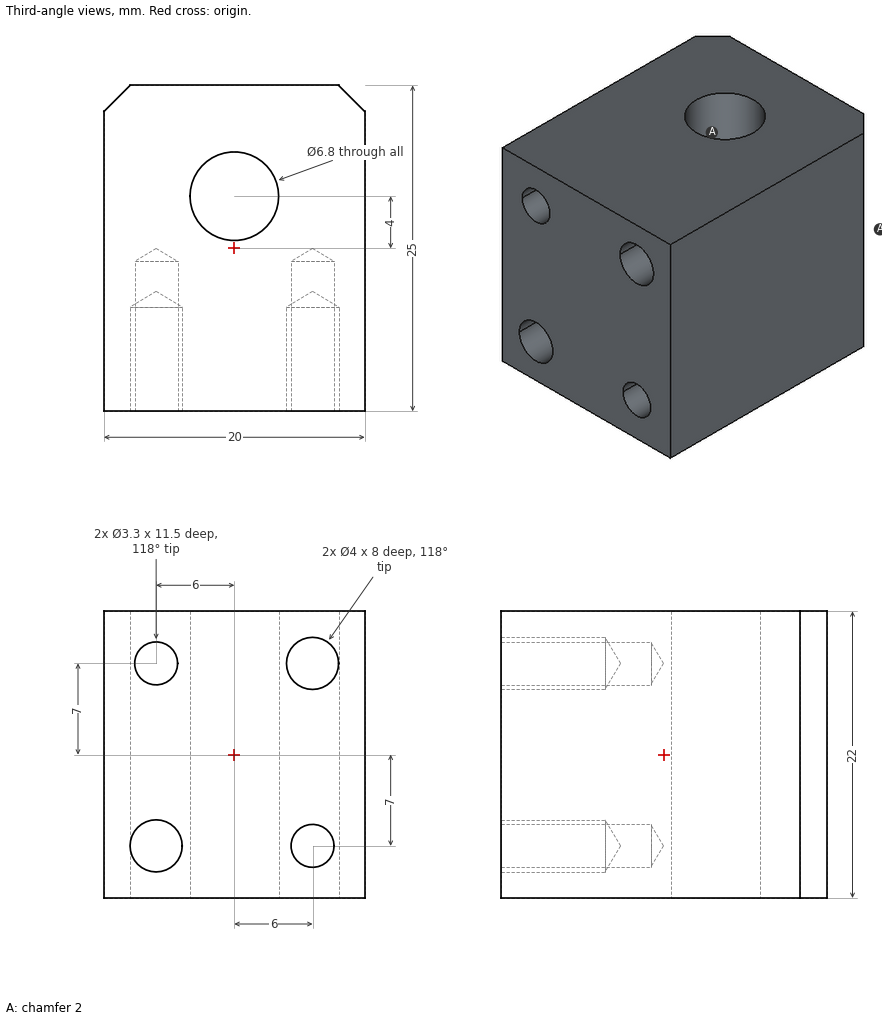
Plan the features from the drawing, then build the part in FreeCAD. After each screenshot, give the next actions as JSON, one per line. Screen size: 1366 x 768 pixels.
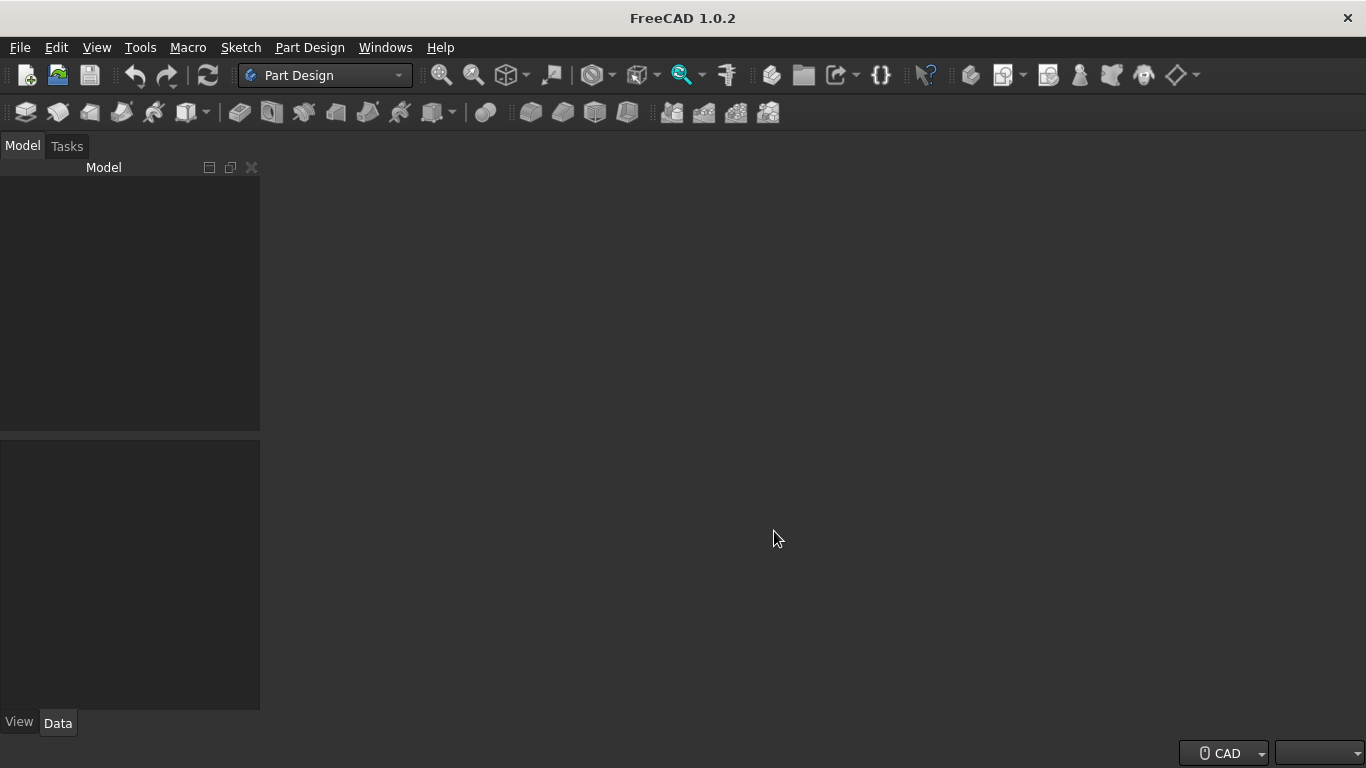
{"action": "left_click", "coordinate": [26, 76]}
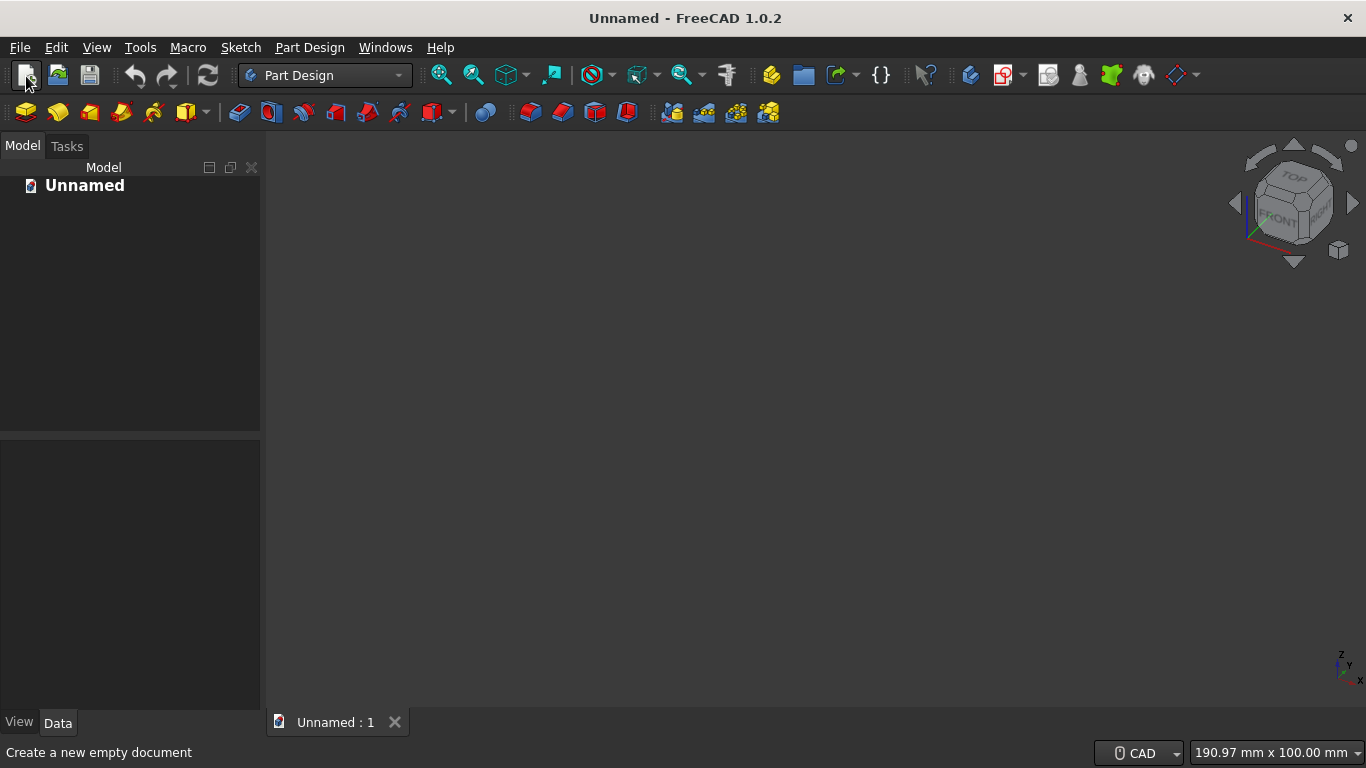
{"action": "left_click", "coordinate": [1004, 76]}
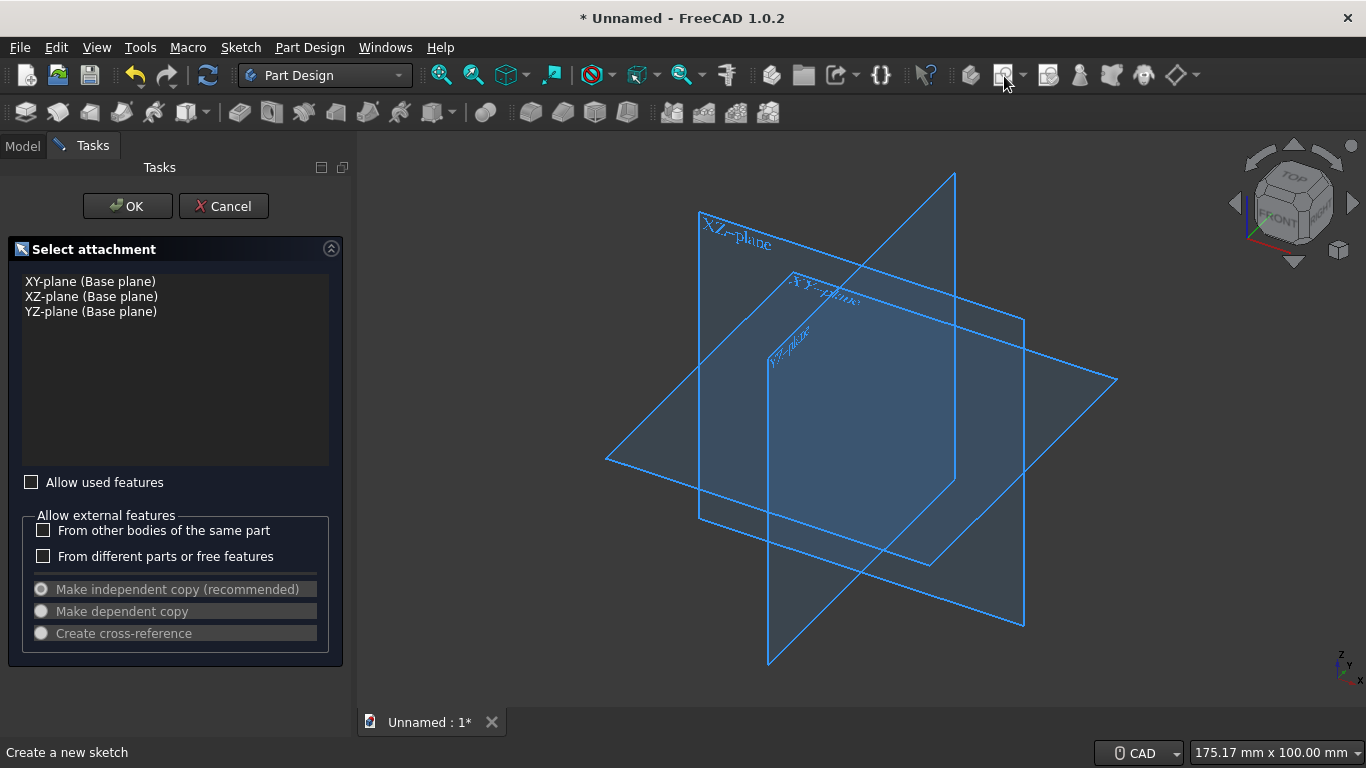
{"action": "left_click", "coordinate": [82, 282]}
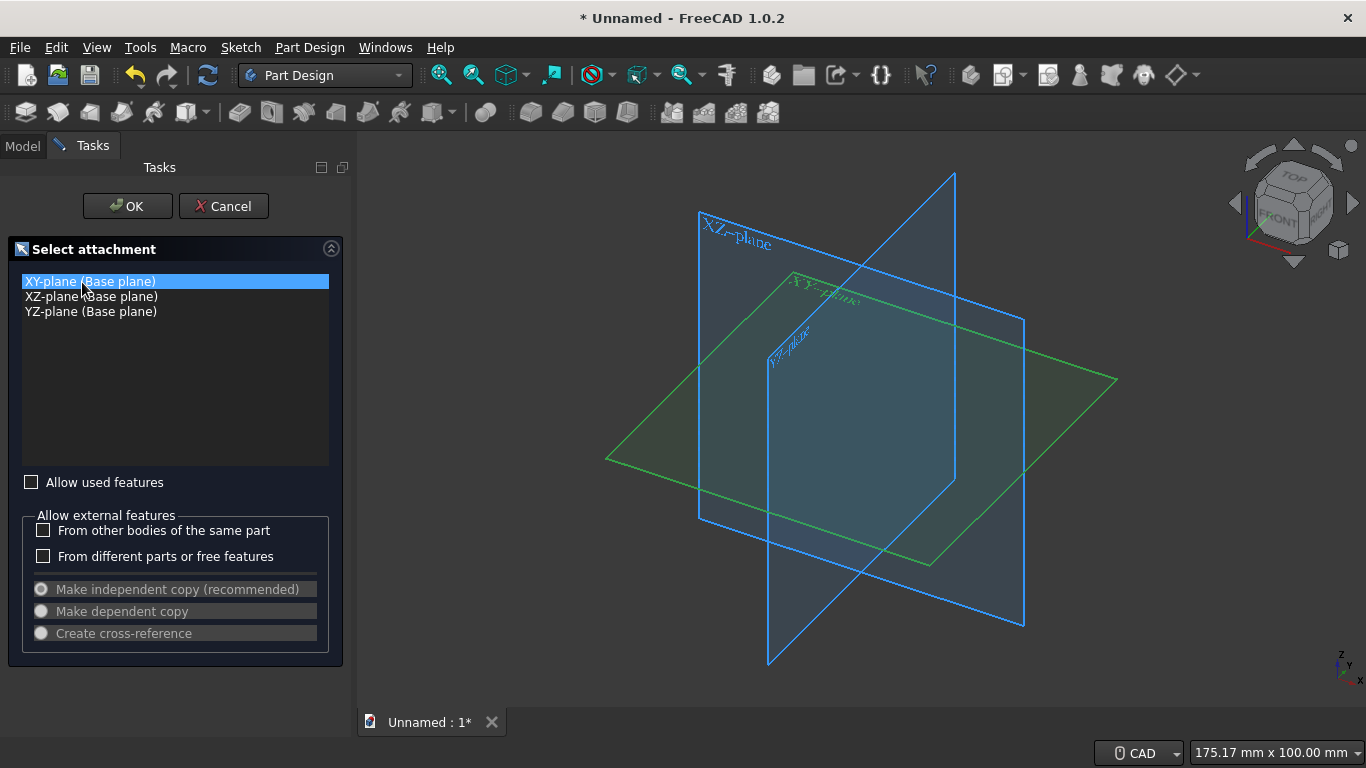
{"action": "left_click", "coordinate": [128, 206]}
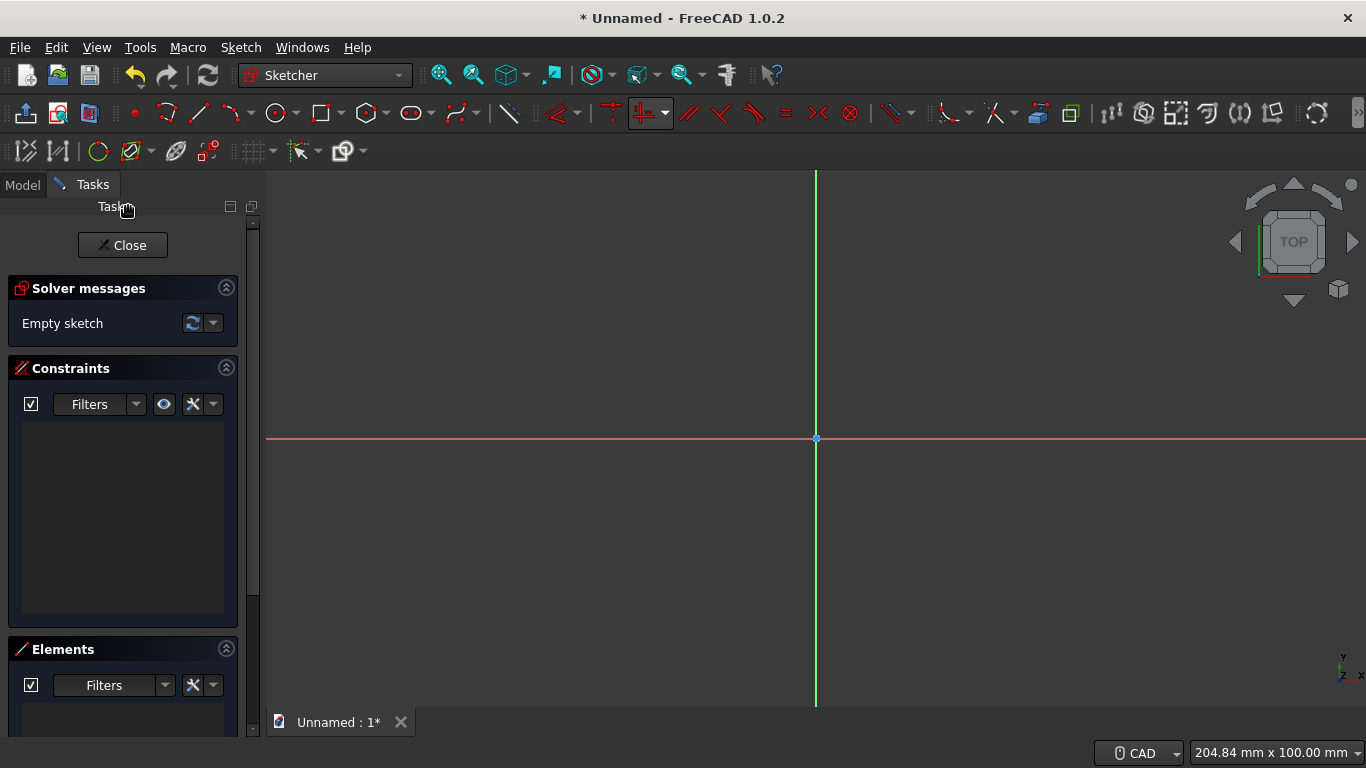
{"action": "scroll", "coordinate": [856, 439], "scroll_direction": "up", "scroll_amount": 5}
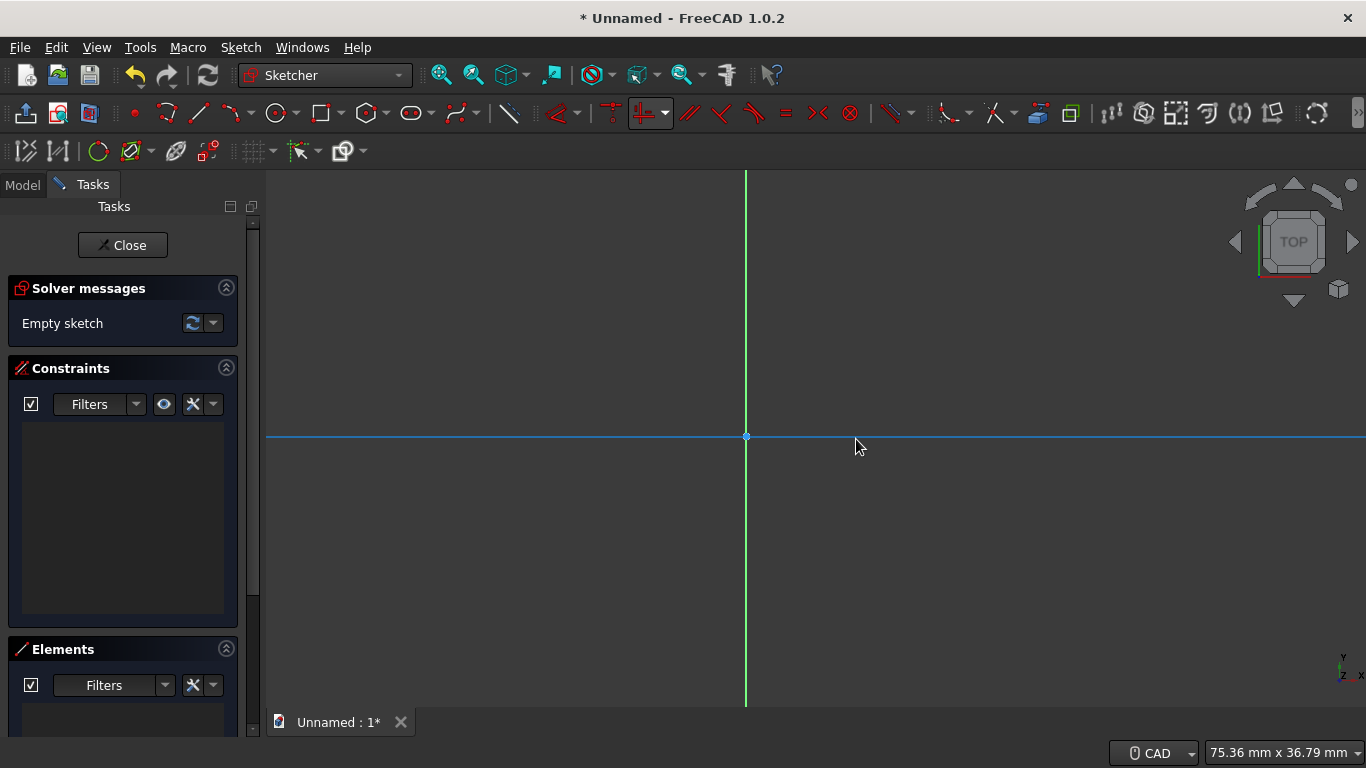
{"action": "left_click", "coordinate": [344, 114]}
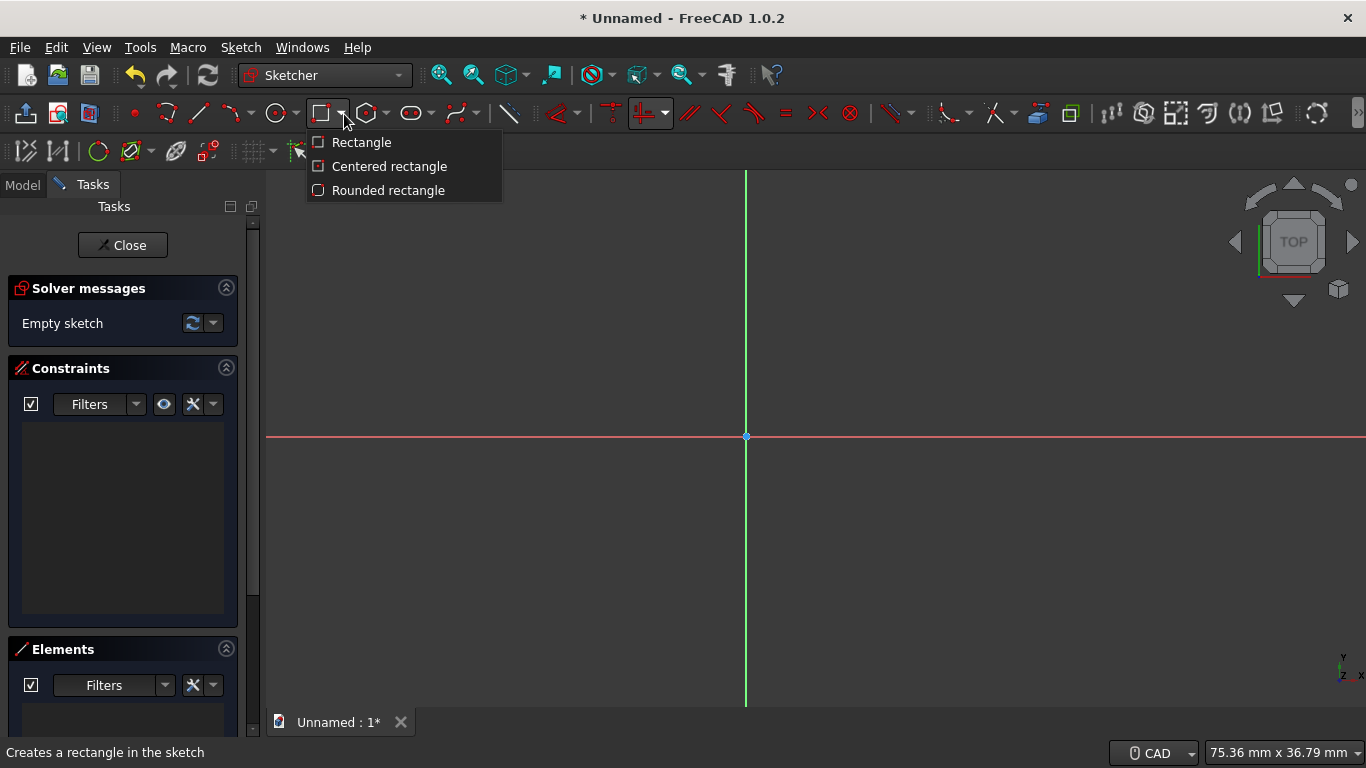
{"action": "left_click", "coordinate": [404, 166]}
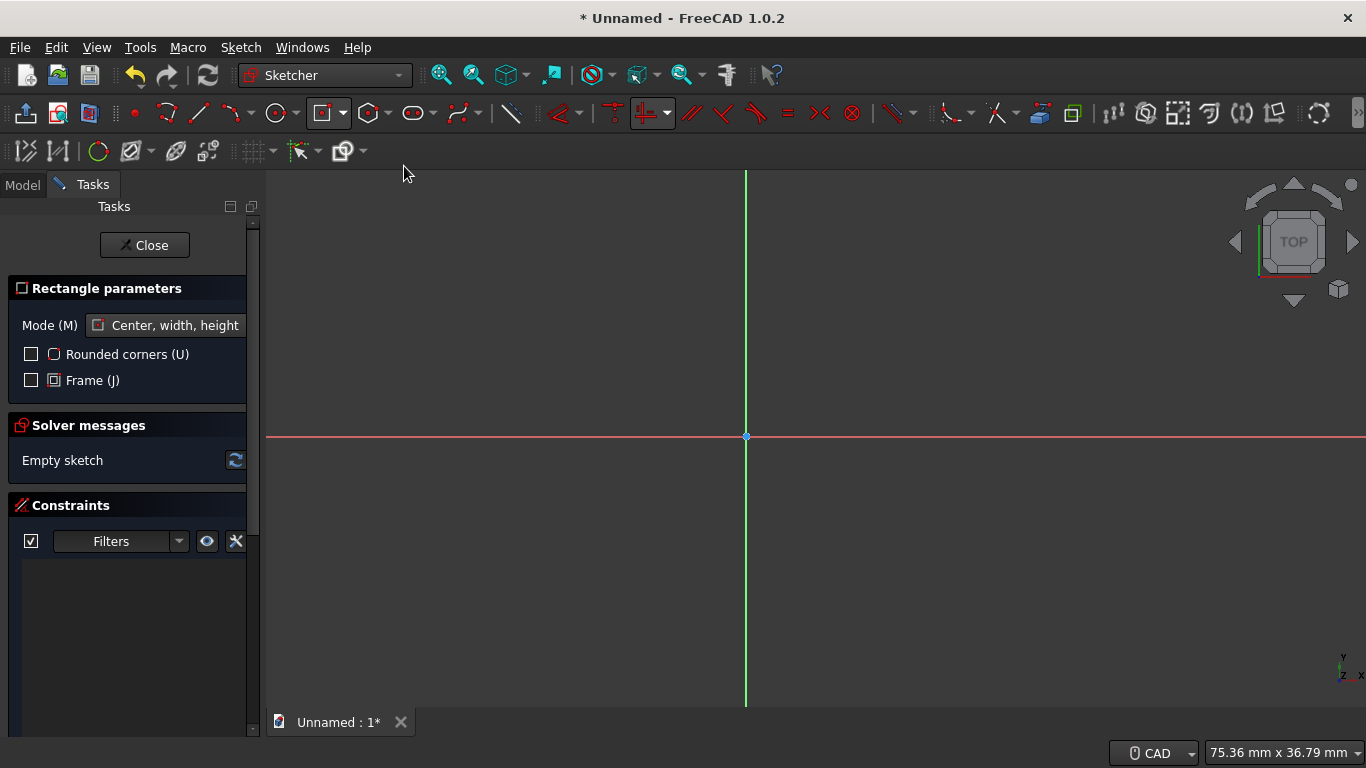
{"action": "left_click", "coordinate": [746, 437]}
{"action": "mouse_move", "coordinate": [892, 254]}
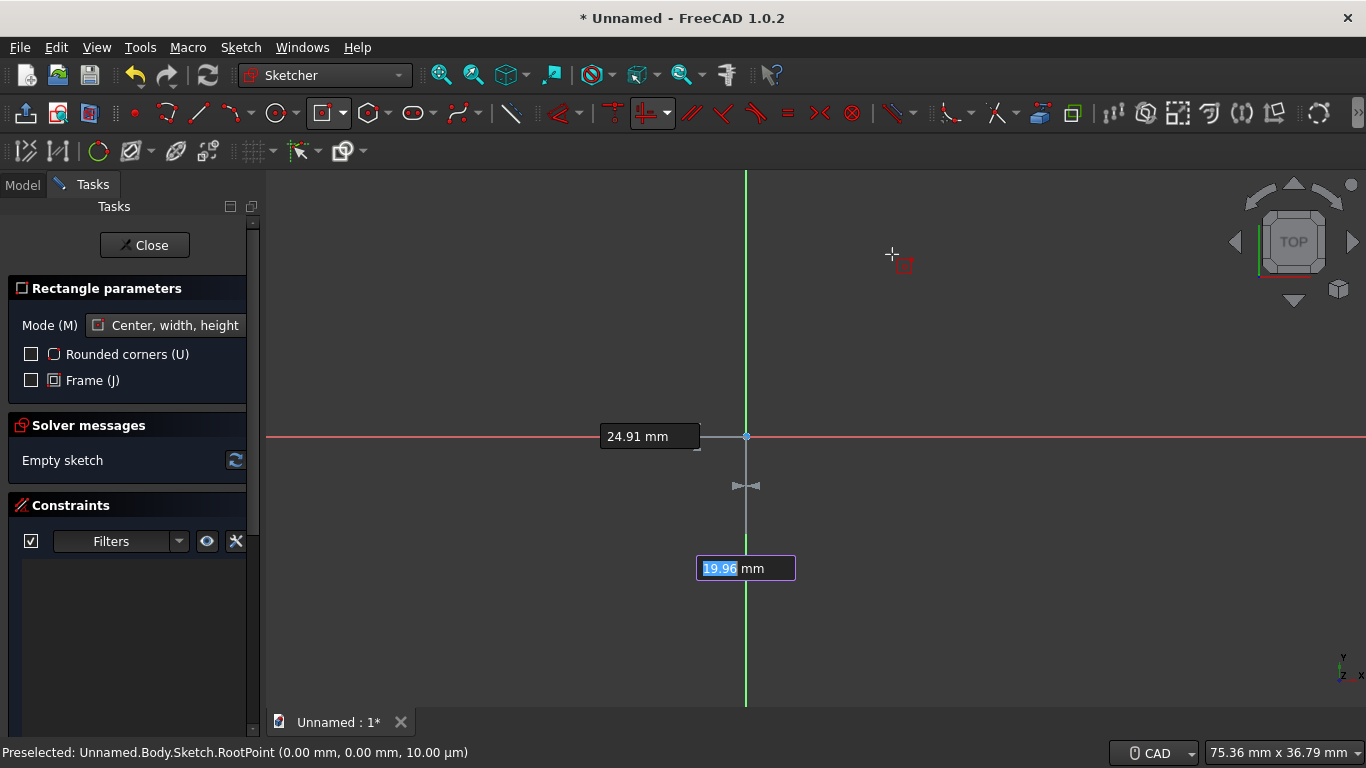
{"action": "type", "text": "20"}
{"action": "key", "text": "Tab"}
{"action": "type", "text": "25"}
{"action": "key", "text": "Return"}
{"action": "key", "text": "Escape"}